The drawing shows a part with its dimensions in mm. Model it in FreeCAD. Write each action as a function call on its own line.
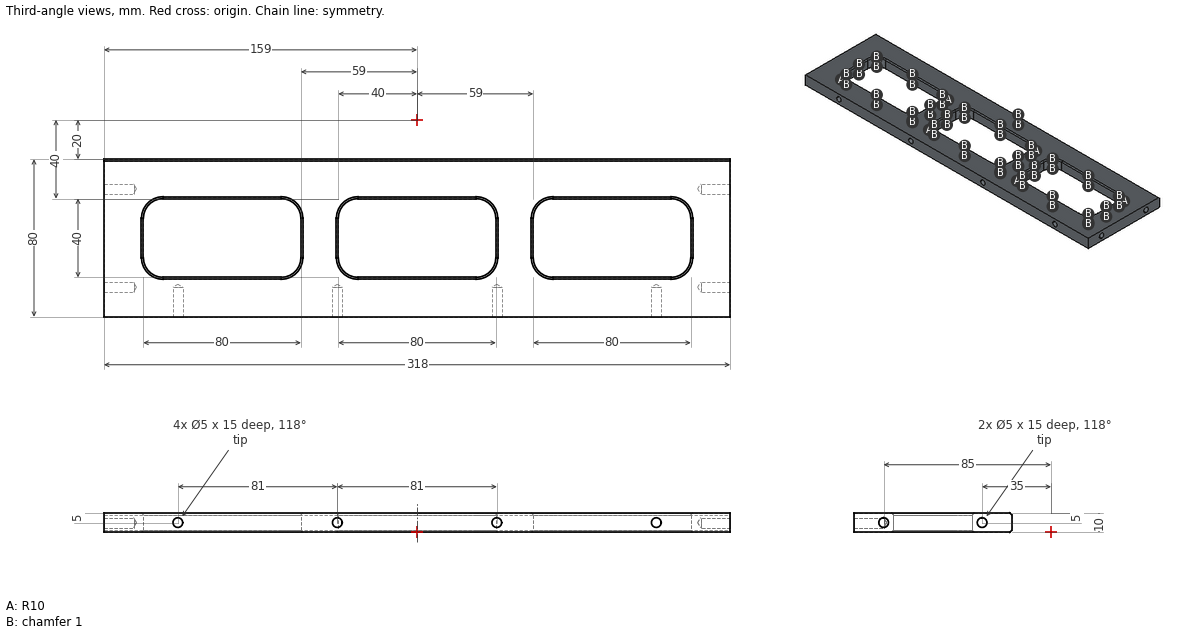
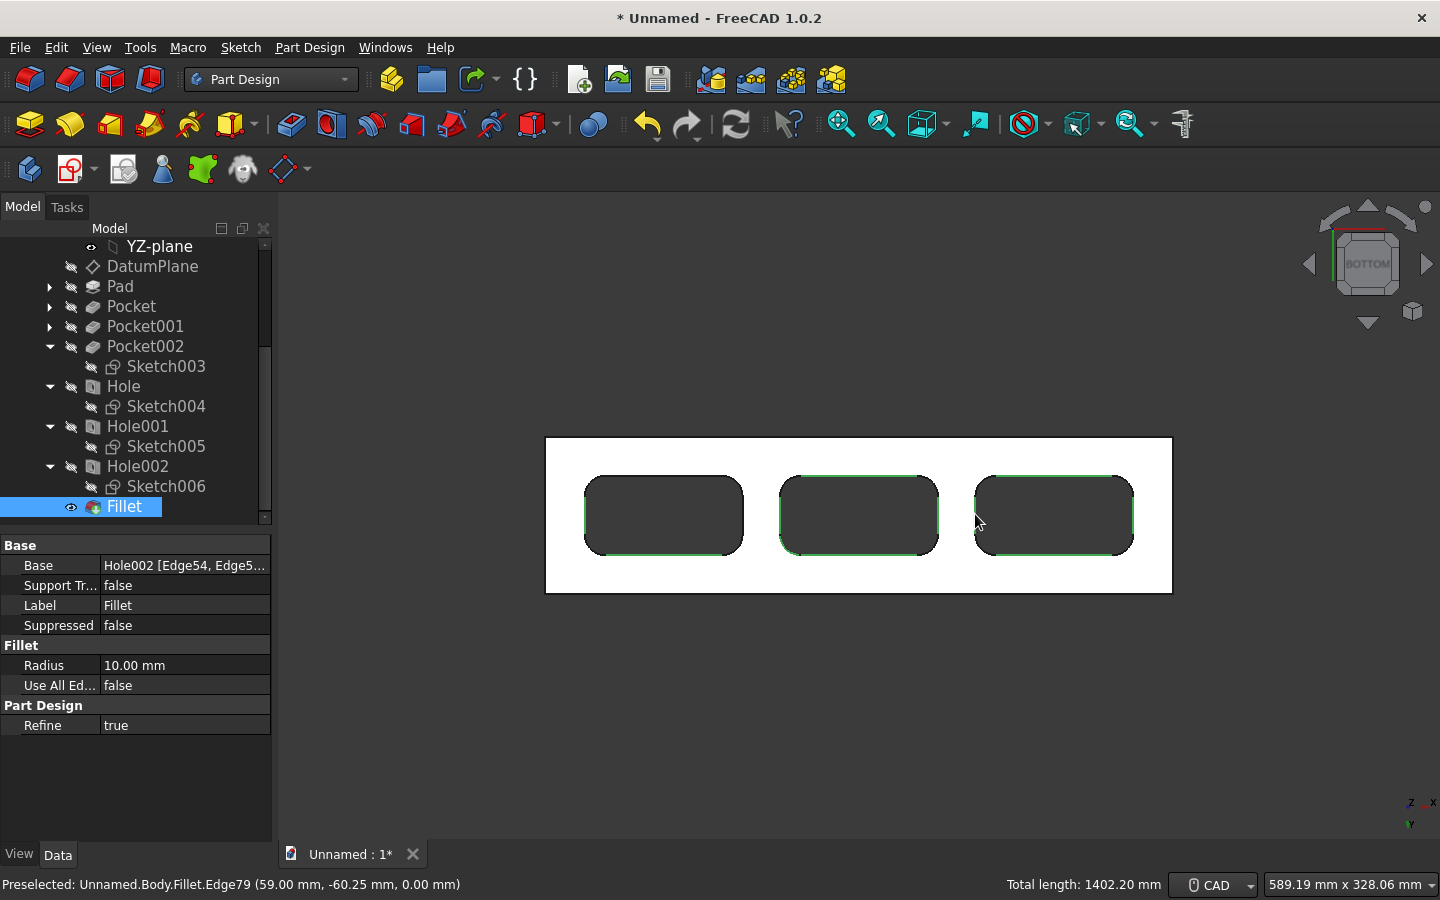
click(743, 514, ctrl)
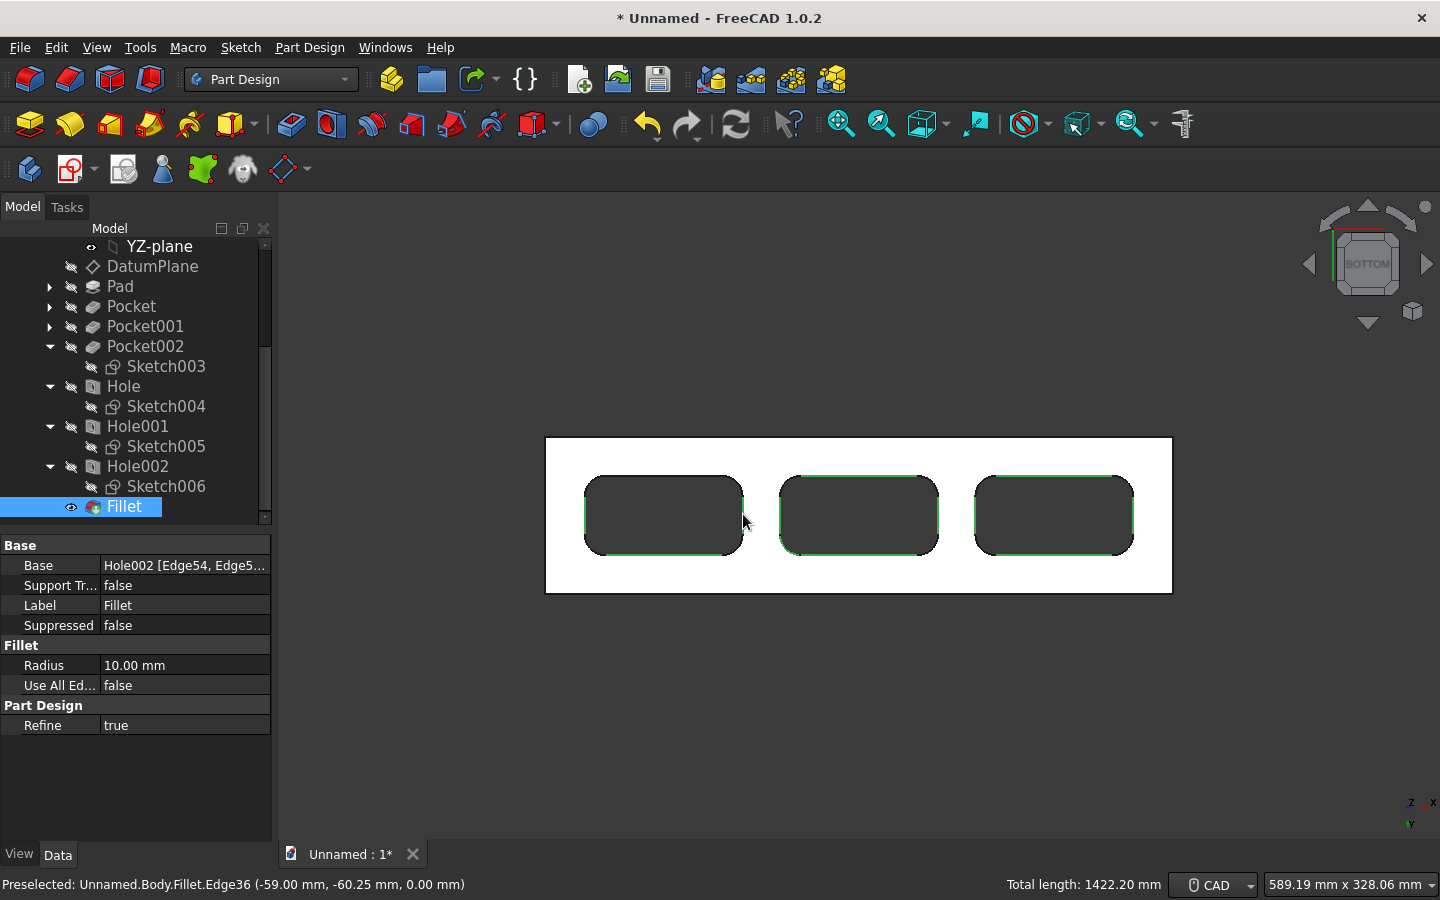
click(664, 475, ctrl)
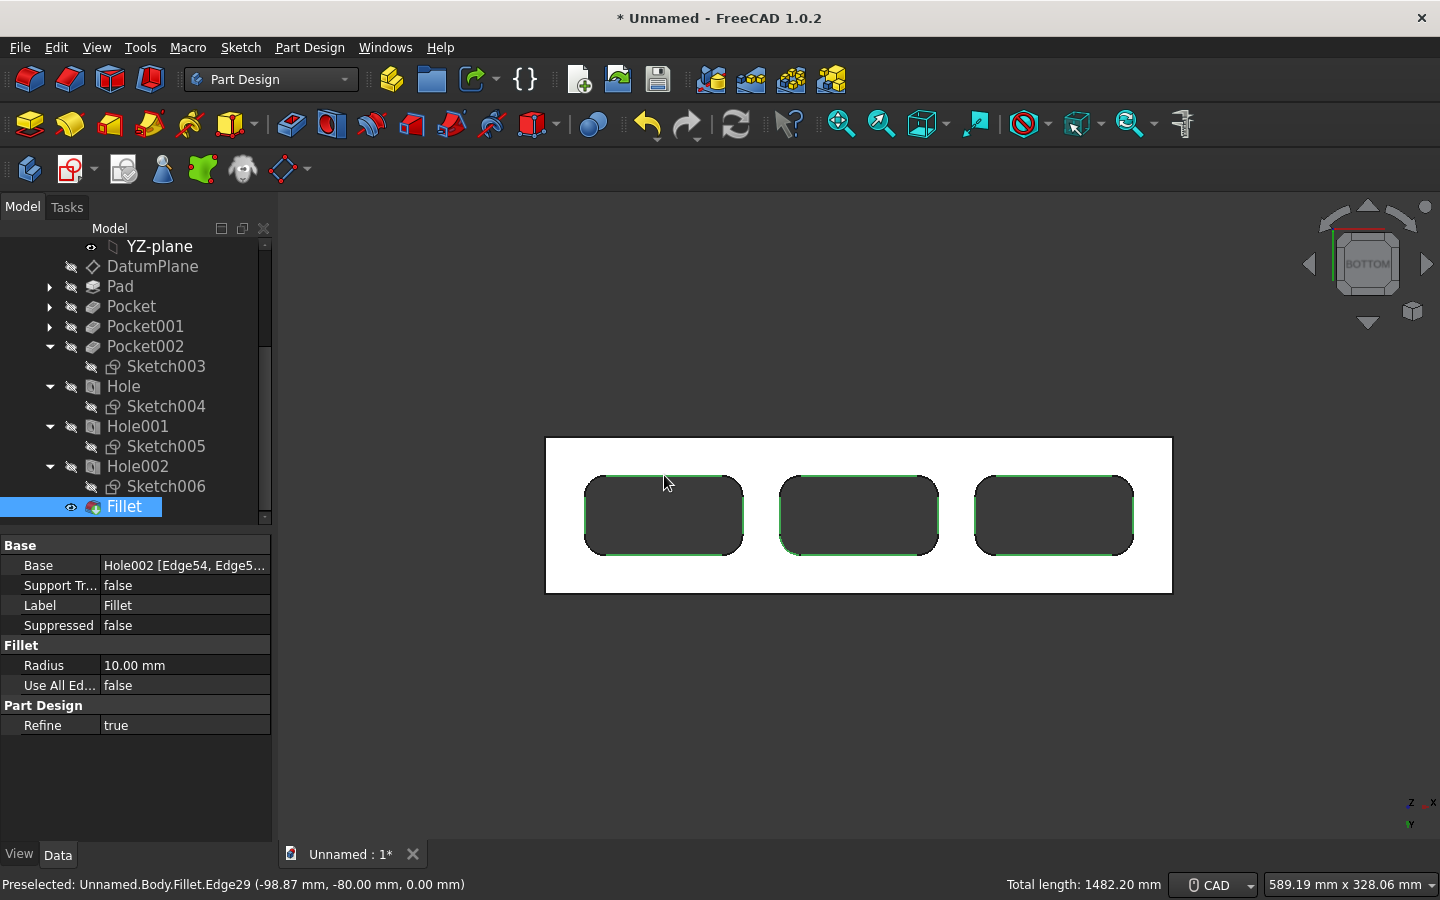
click(932, 548, ctrl)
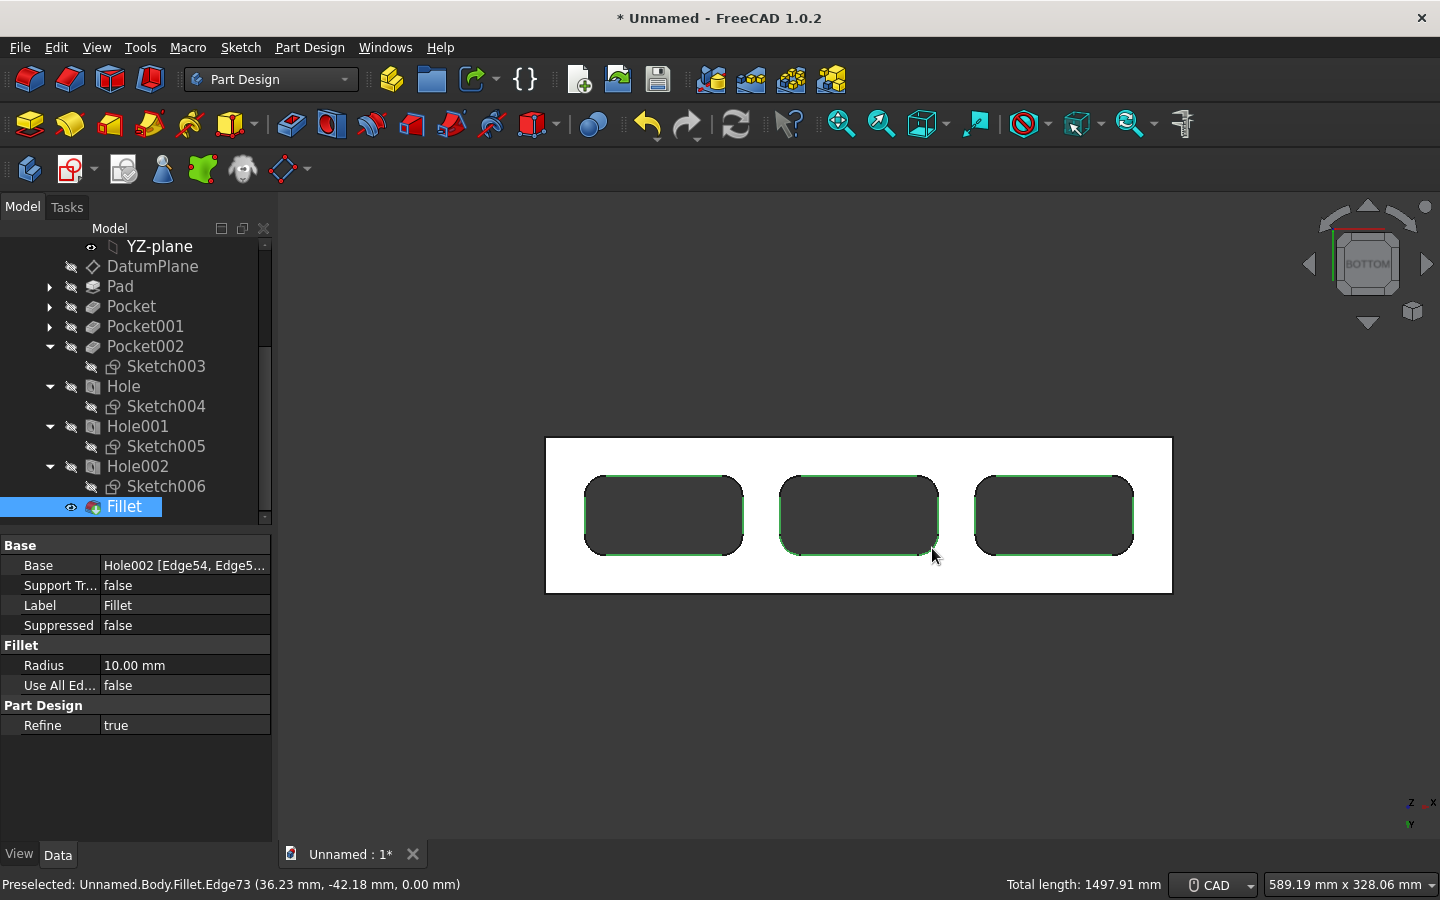
click(1127, 548, ctrl)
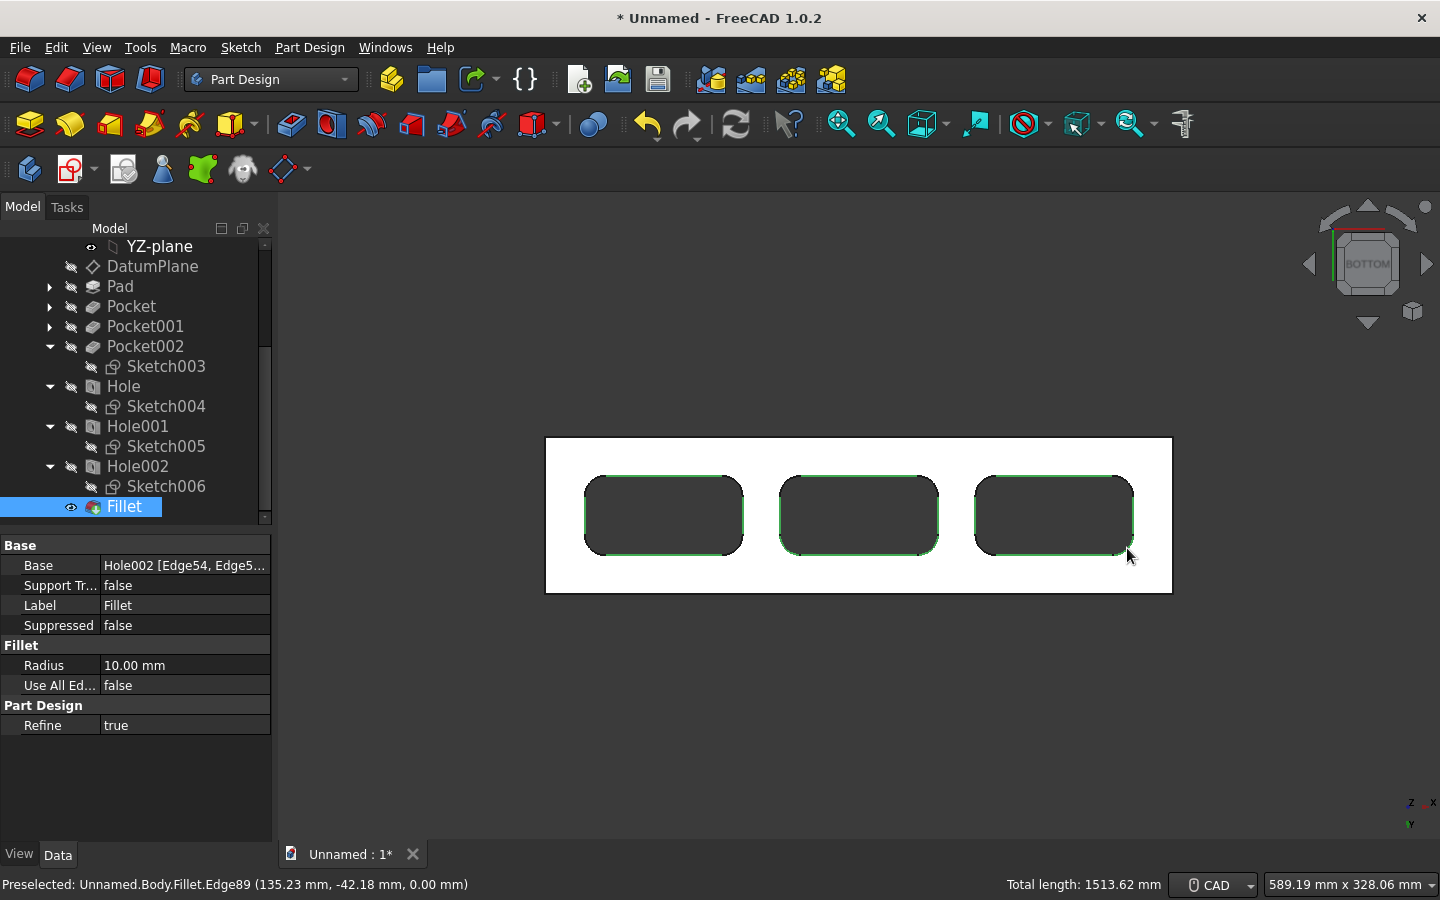
click(786, 481, ctrl)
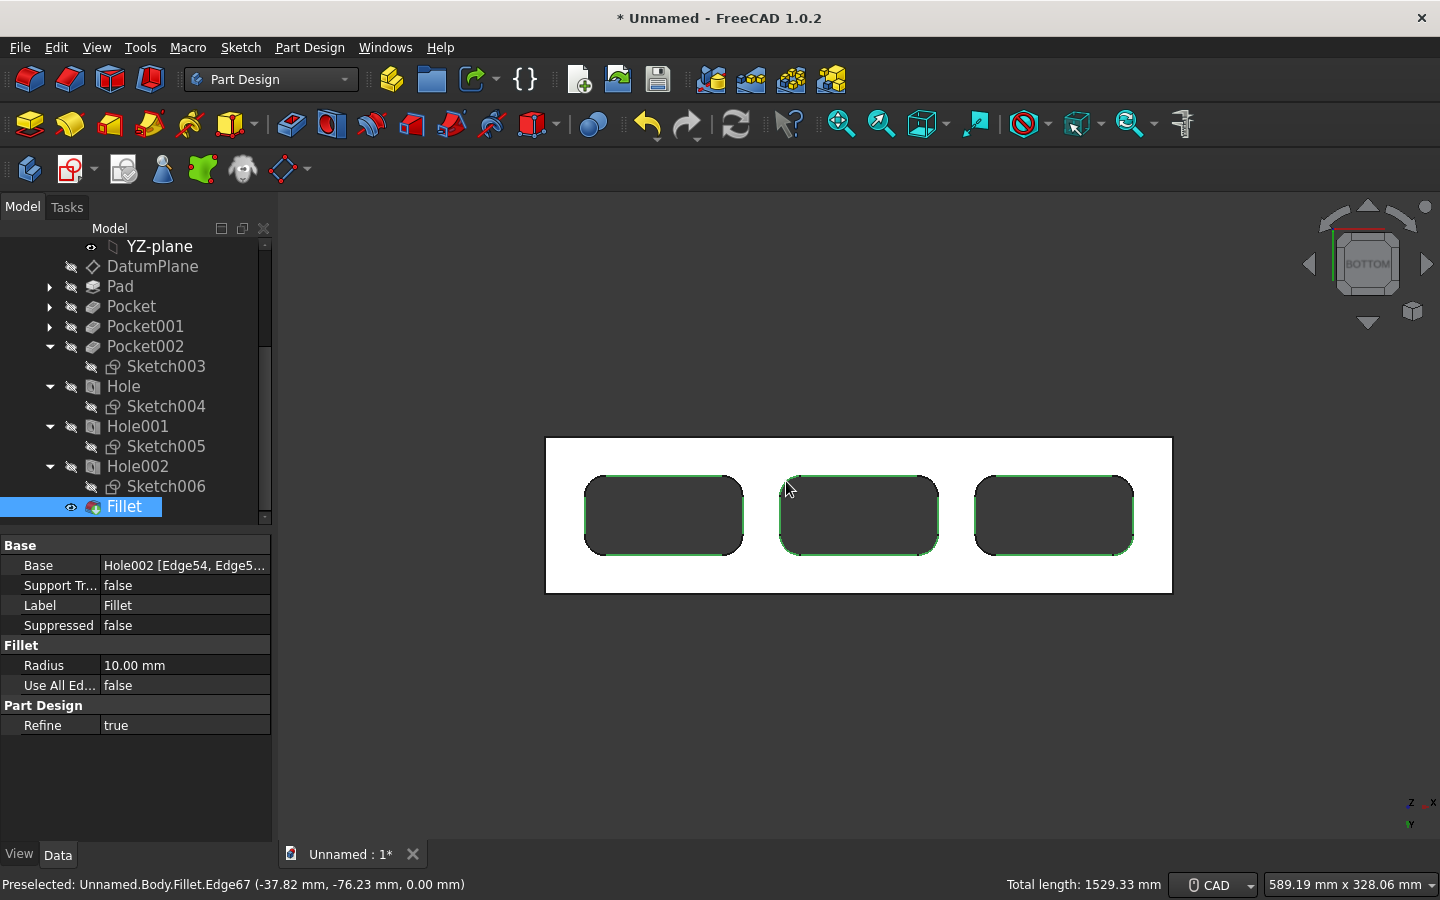
click(1127, 481, ctrl)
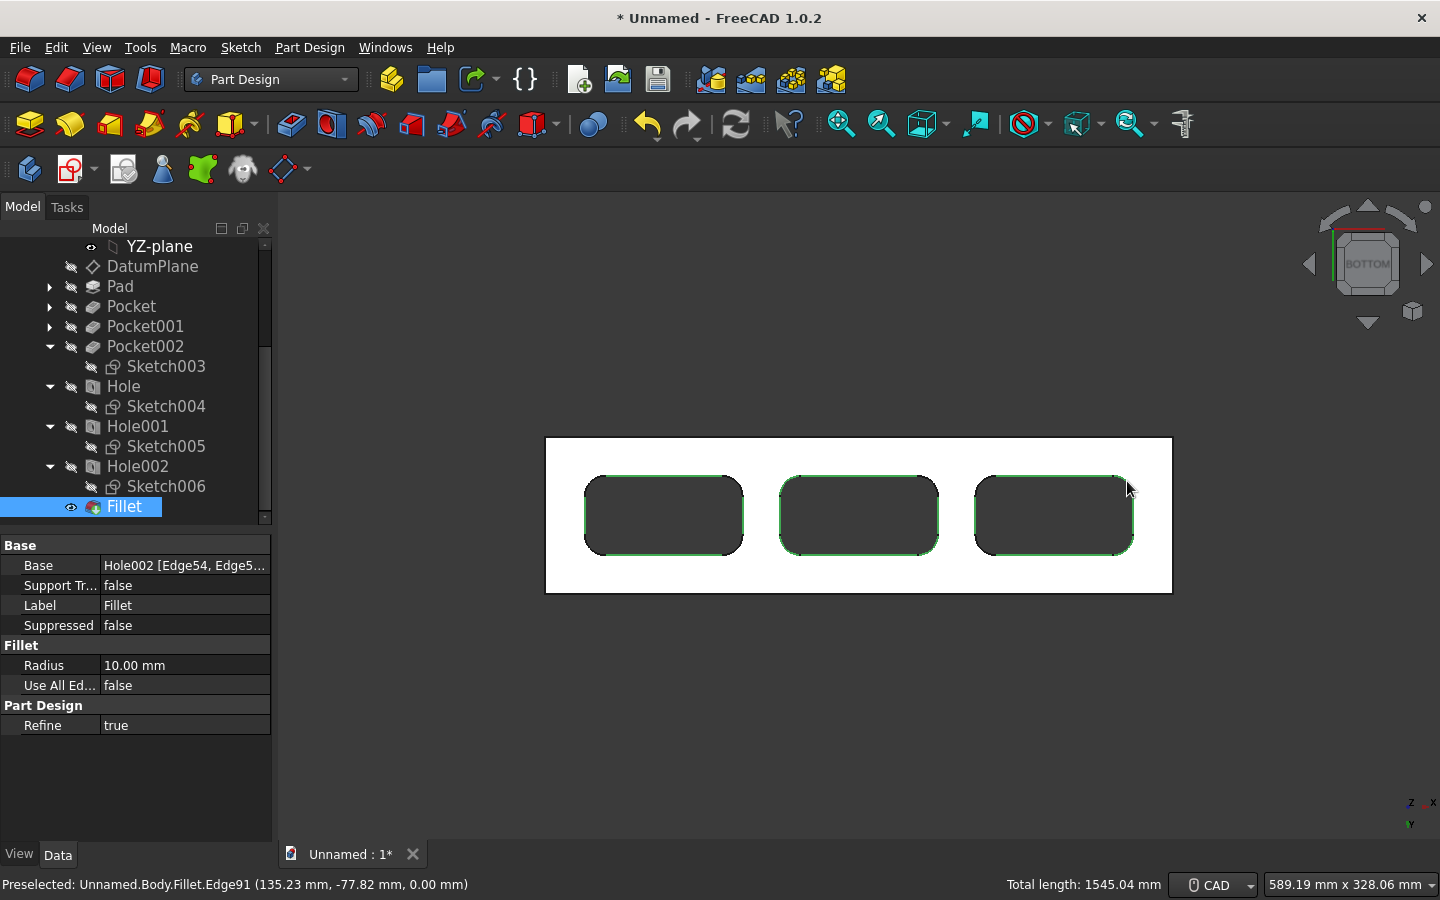
click(591, 548, ctrl)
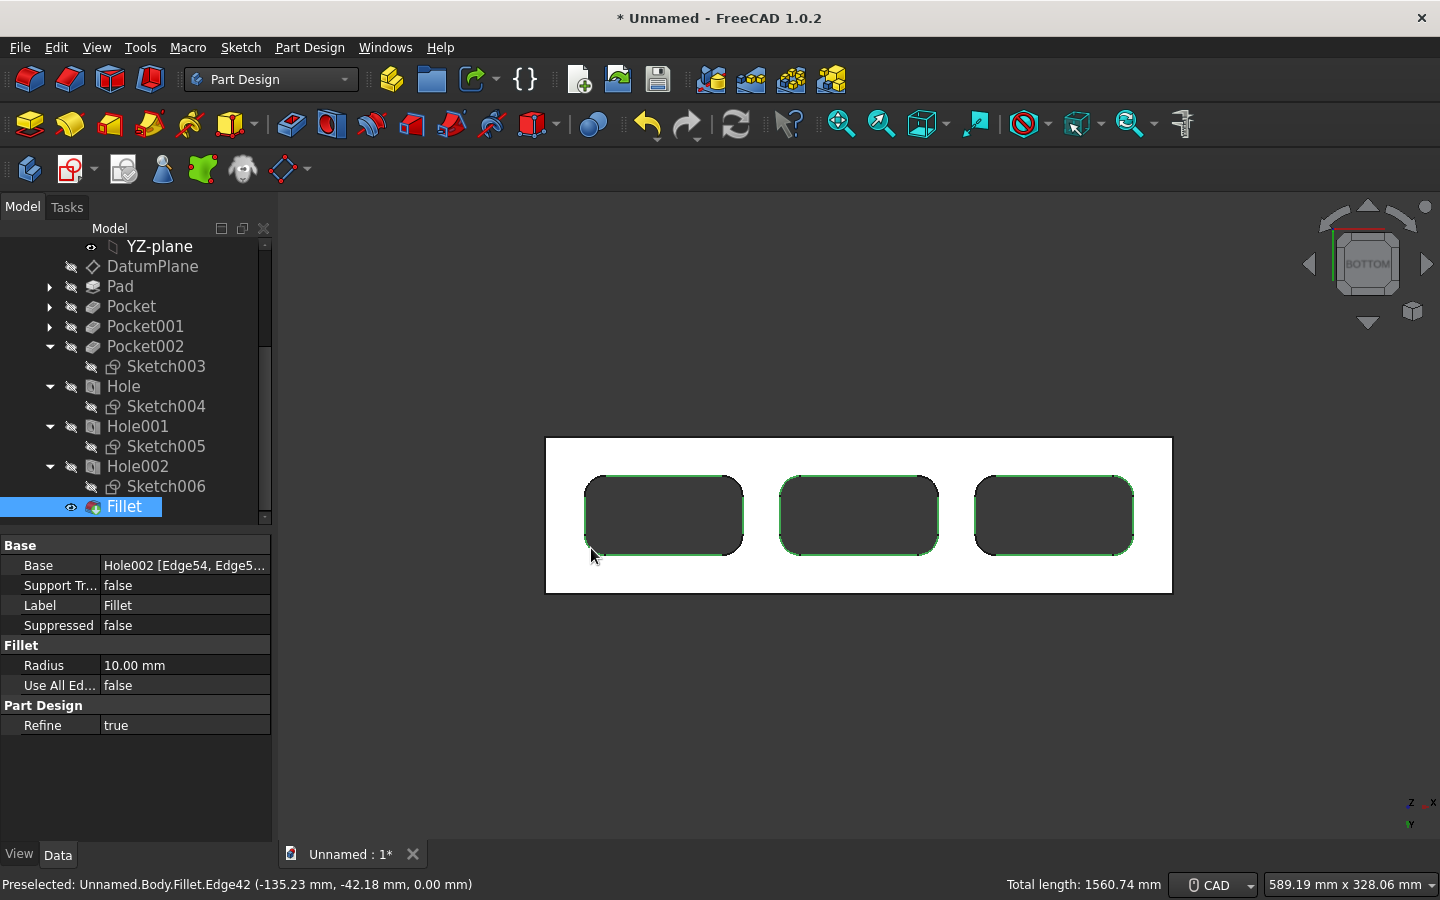
click(981, 548, ctrl)